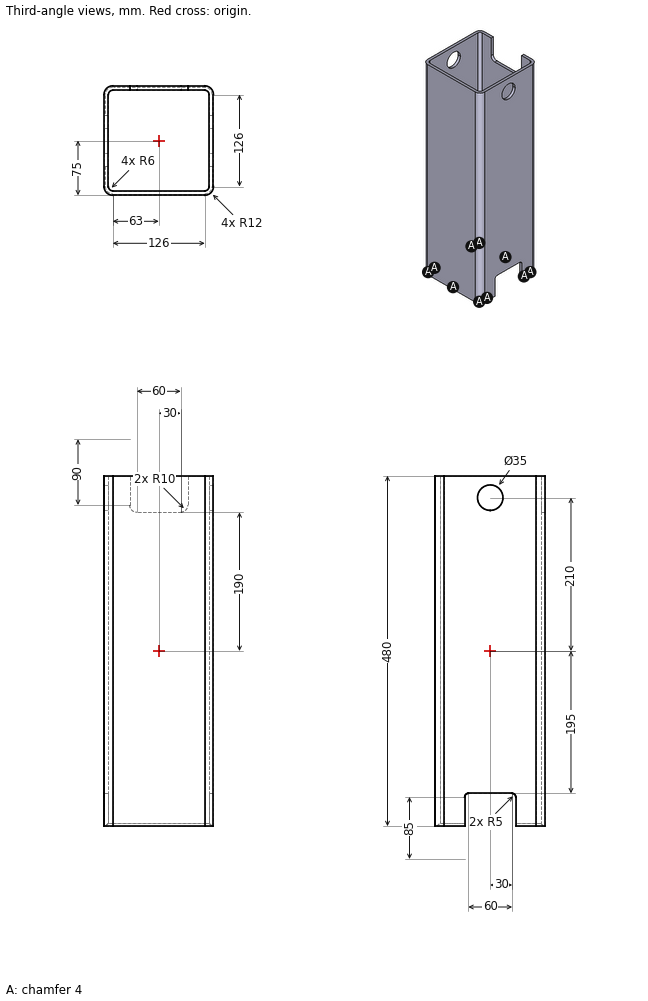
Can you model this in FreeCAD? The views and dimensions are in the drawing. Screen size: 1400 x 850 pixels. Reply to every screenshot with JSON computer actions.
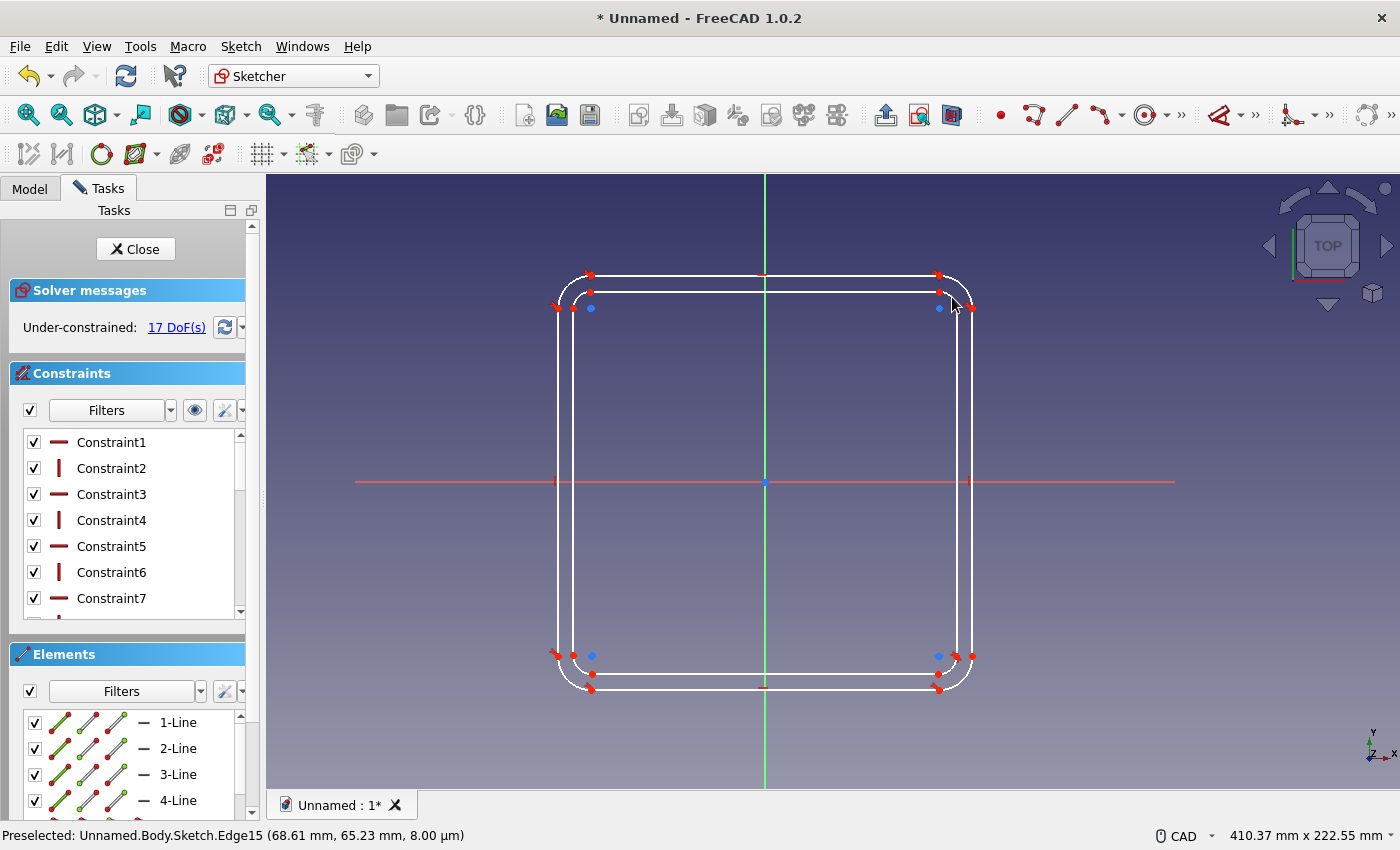
{"action": "left_click", "coordinate": [957, 413]}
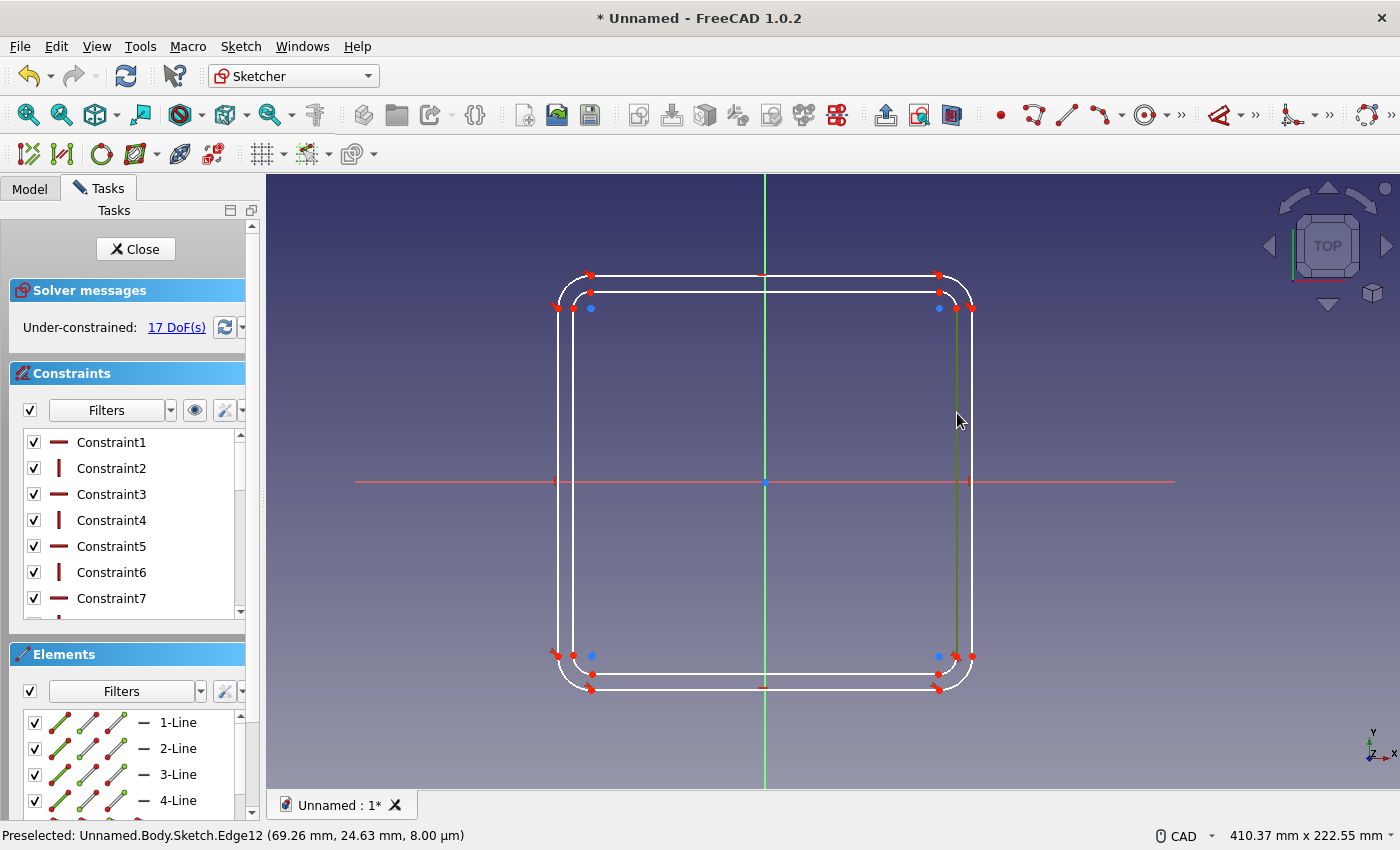
{"action": "left_click", "coordinate": [951, 669]}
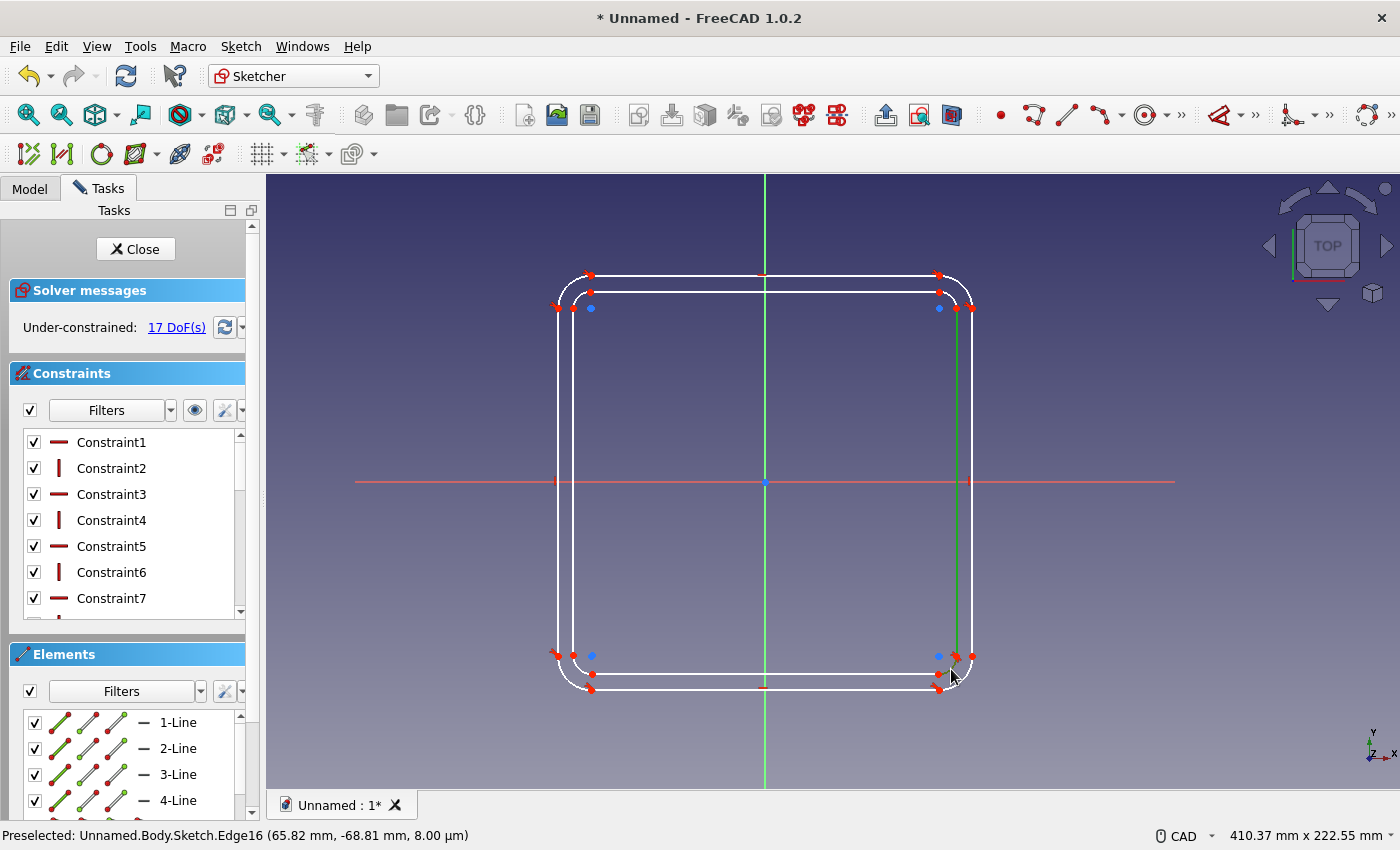
{"action": "key", "text": "t"}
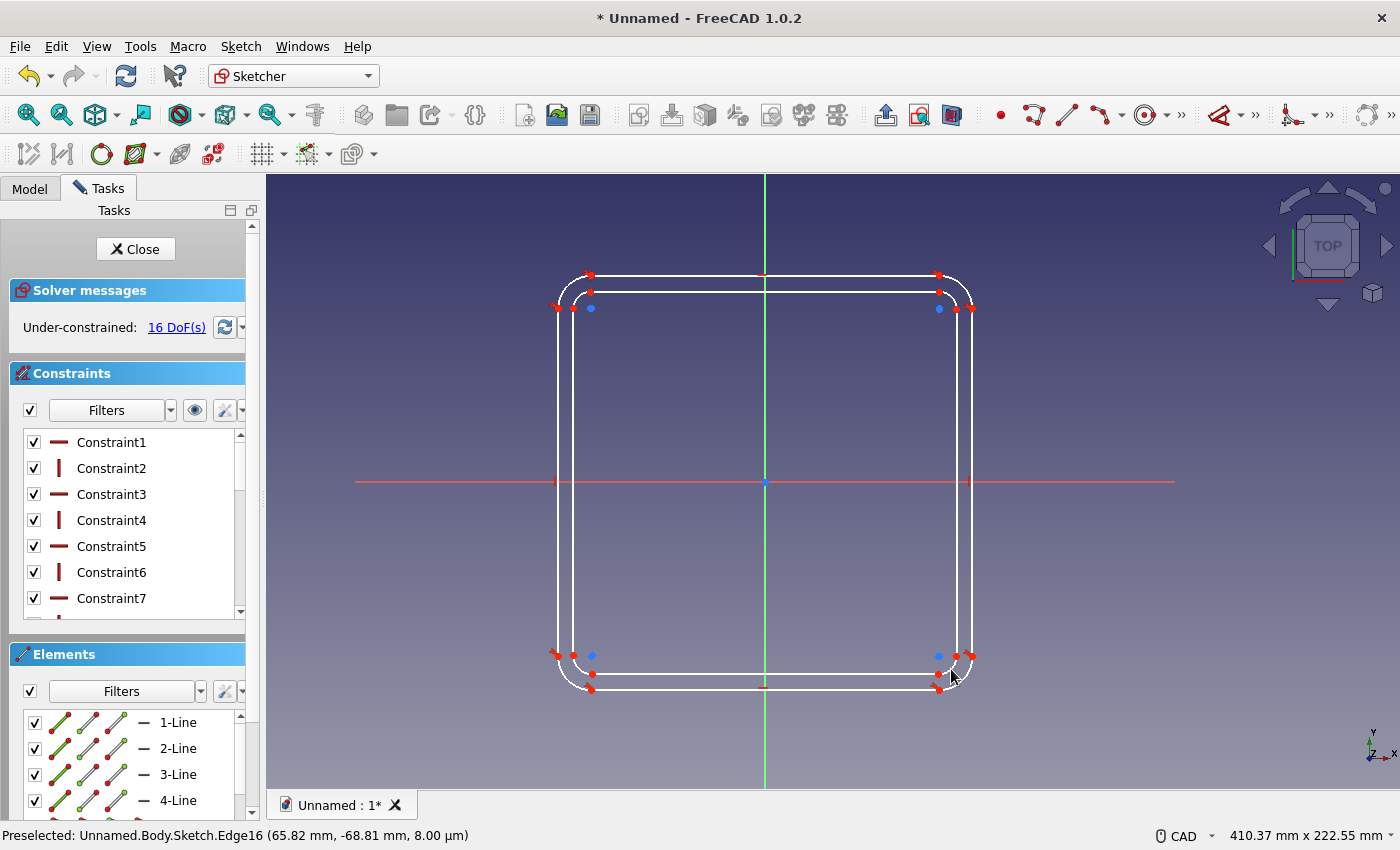
{"action": "left_click", "coordinate": [562, 672]}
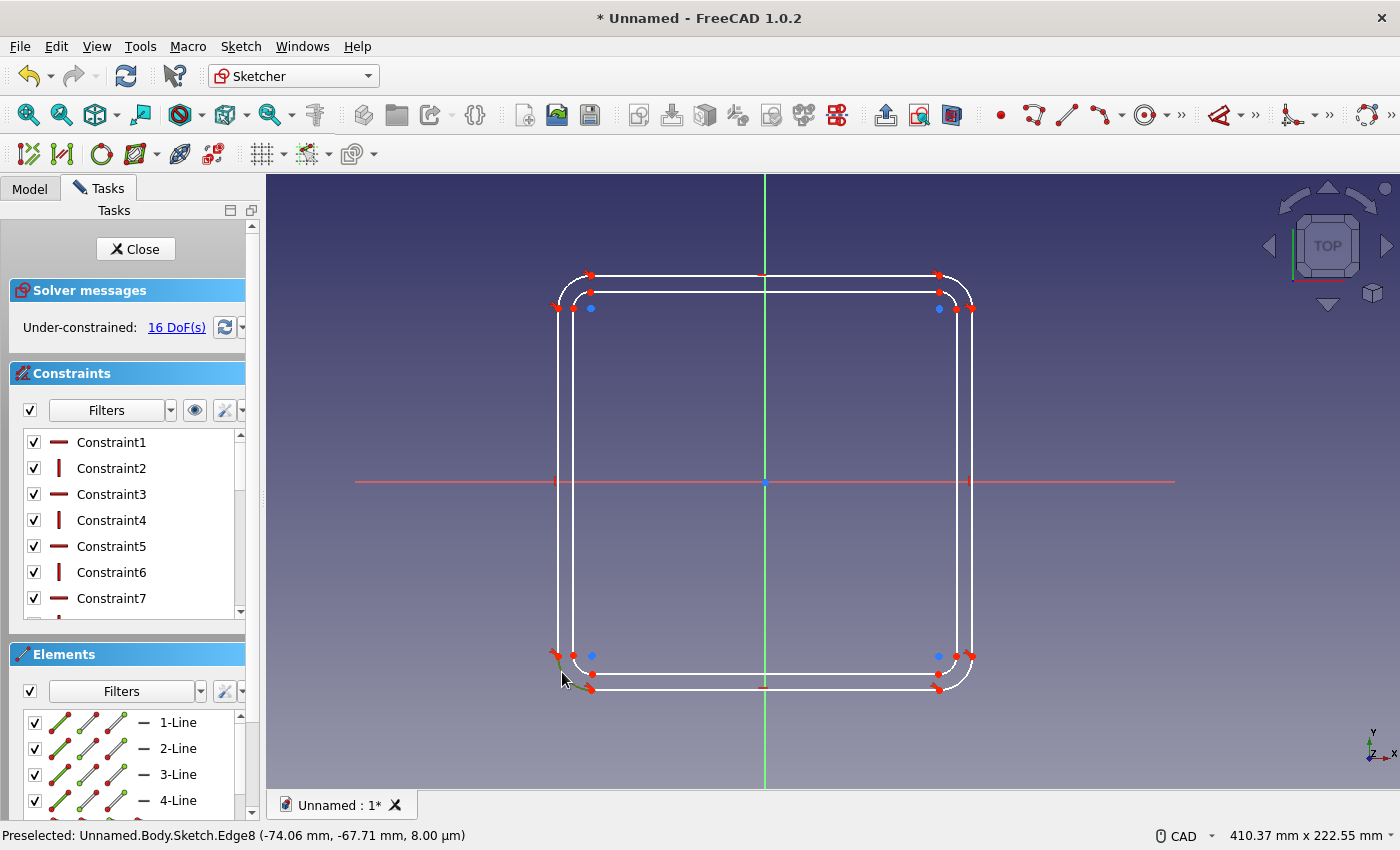
{"action": "left_click", "coordinate": [579, 669]}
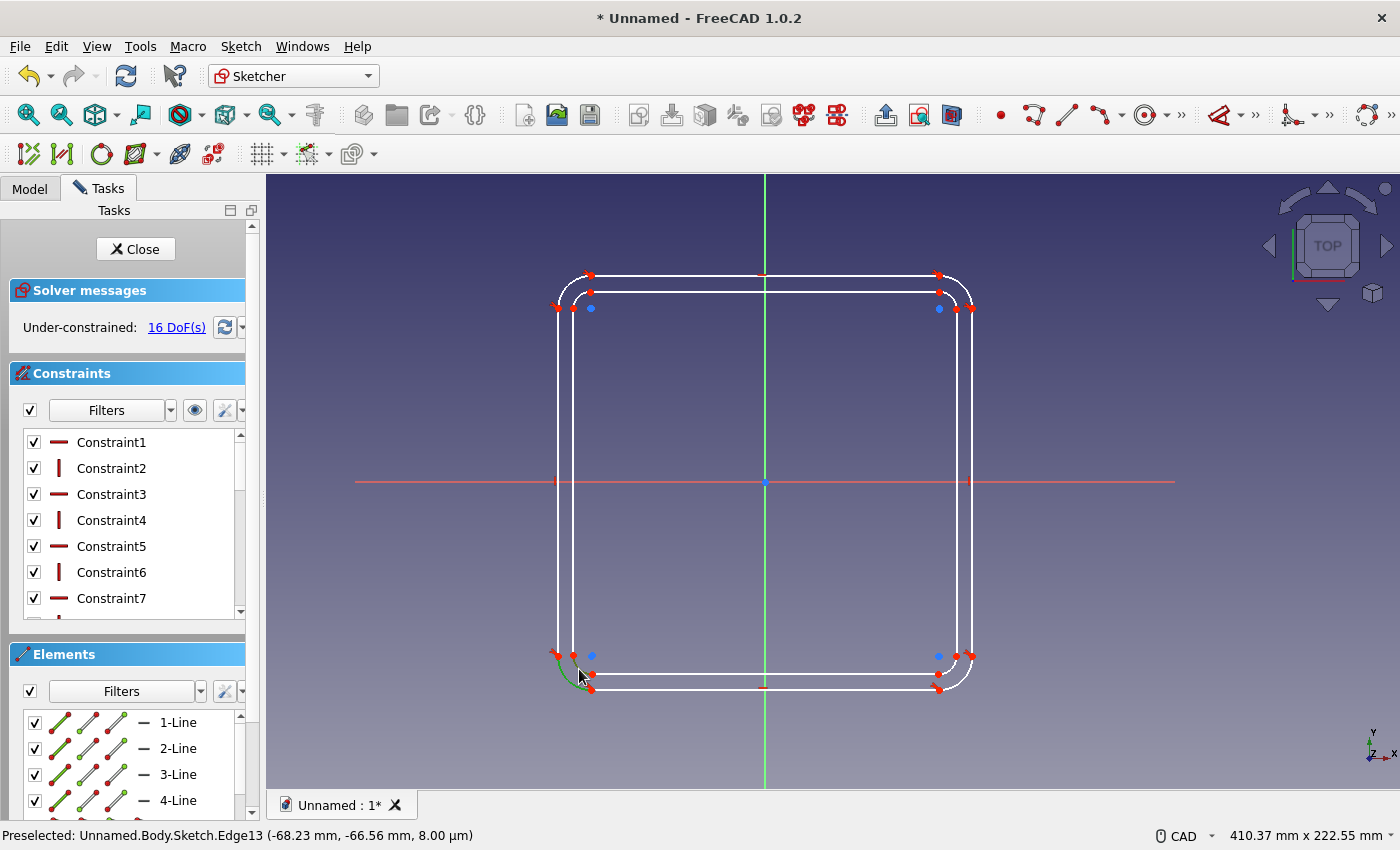
{"action": "key", "text": "c"}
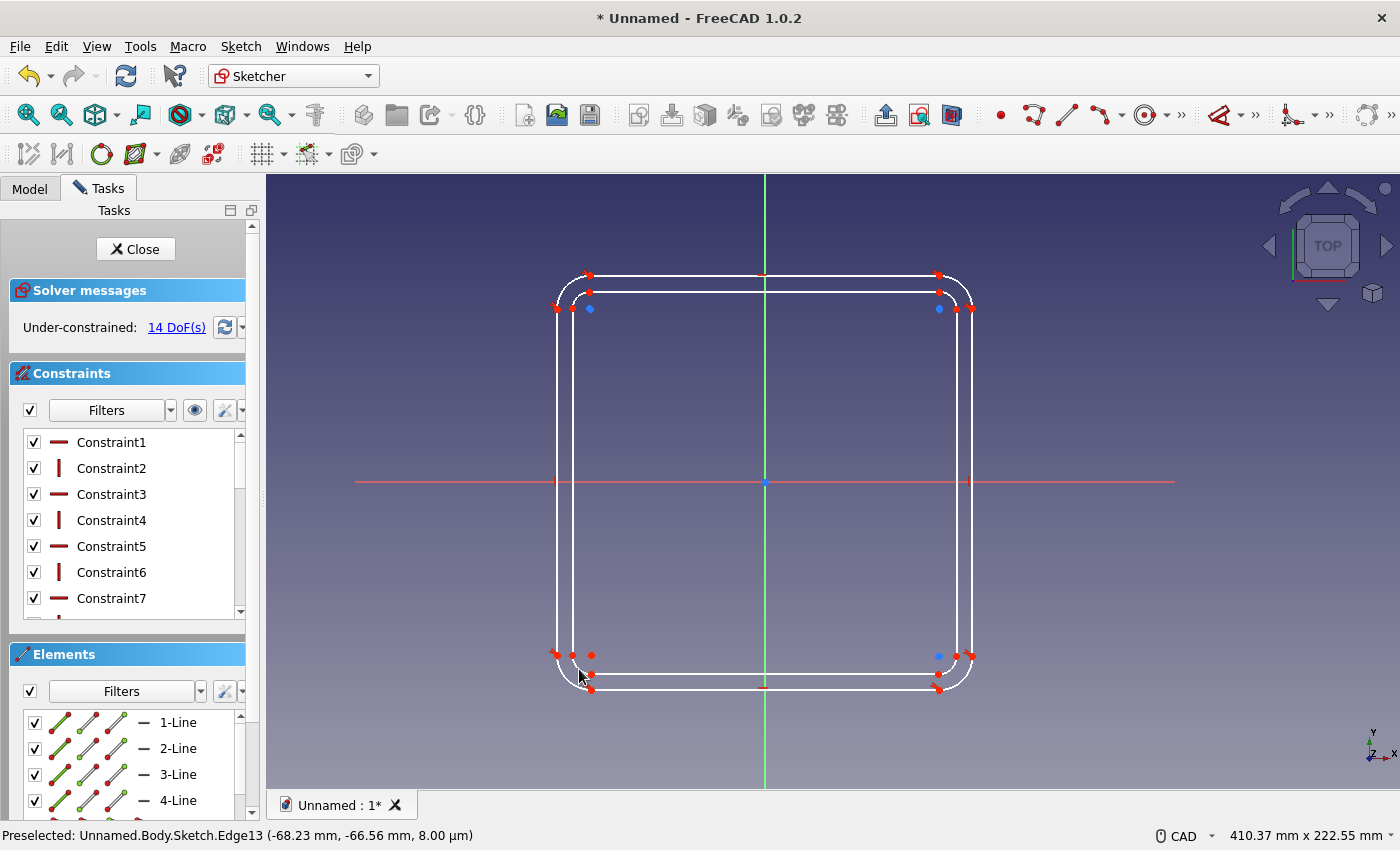
{"action": "left_click", "coordinate": [575, 280]}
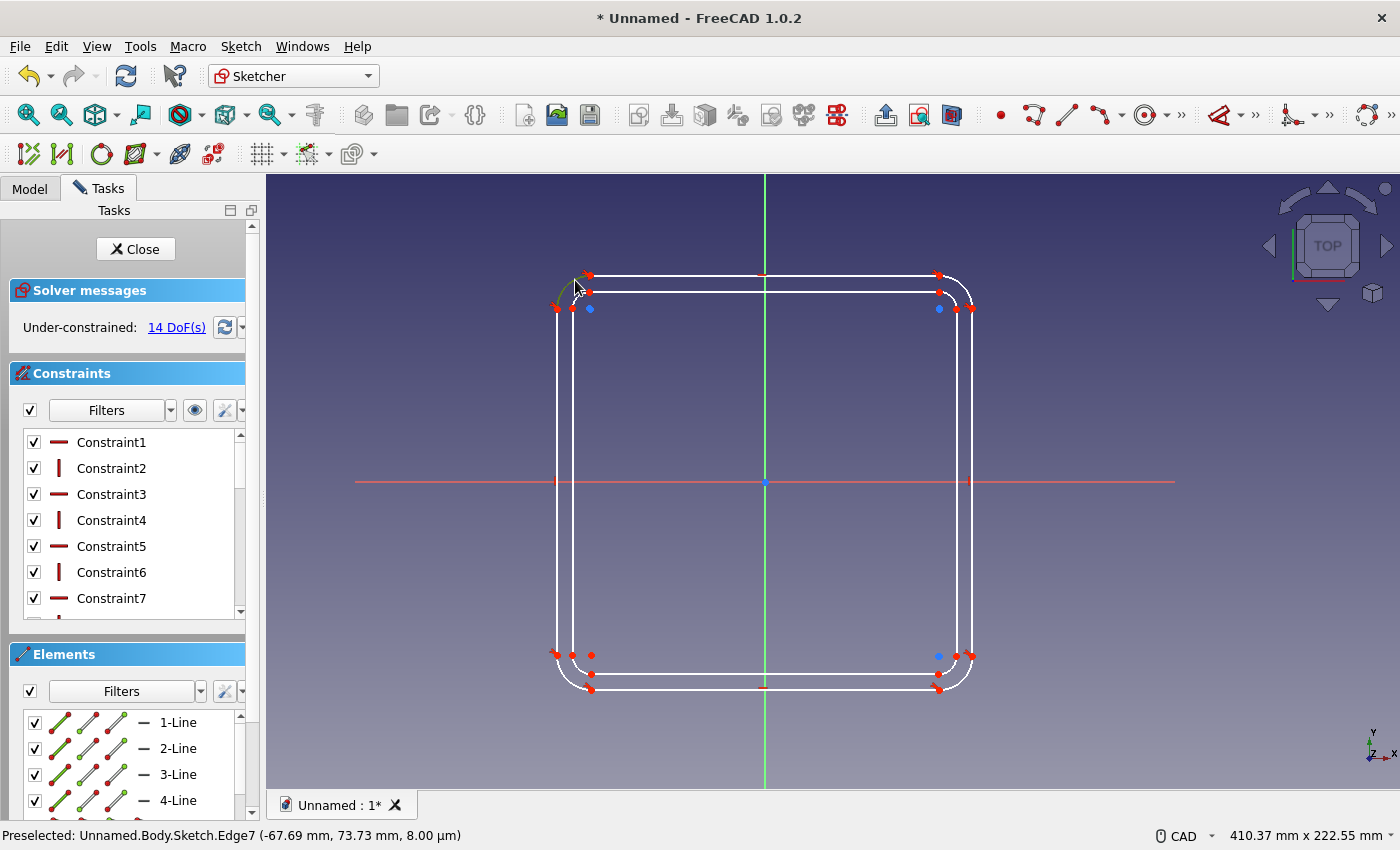
{"action": "left_click", "coordinate": [578, 297]}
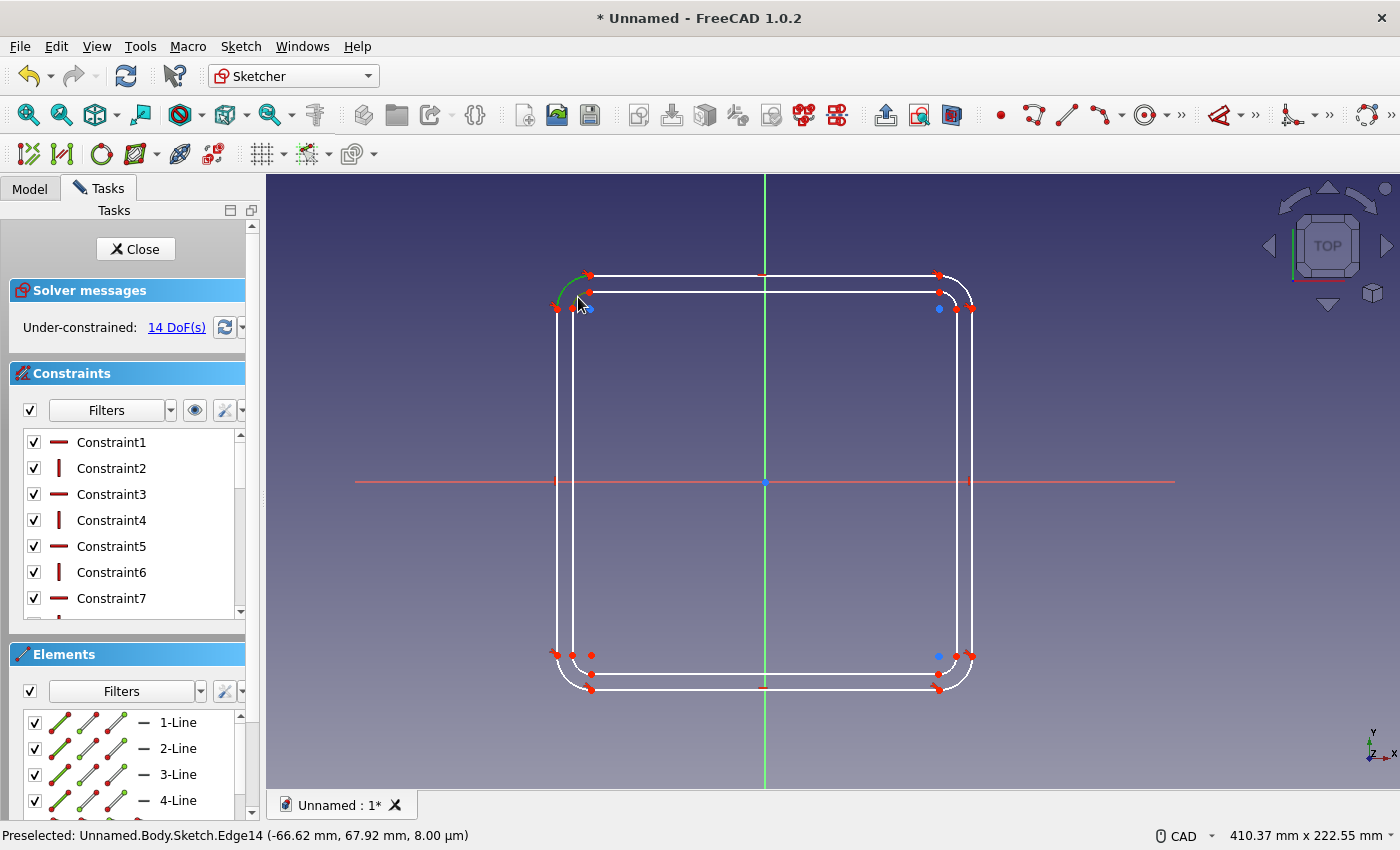
{"action": "key", "text": "c"}